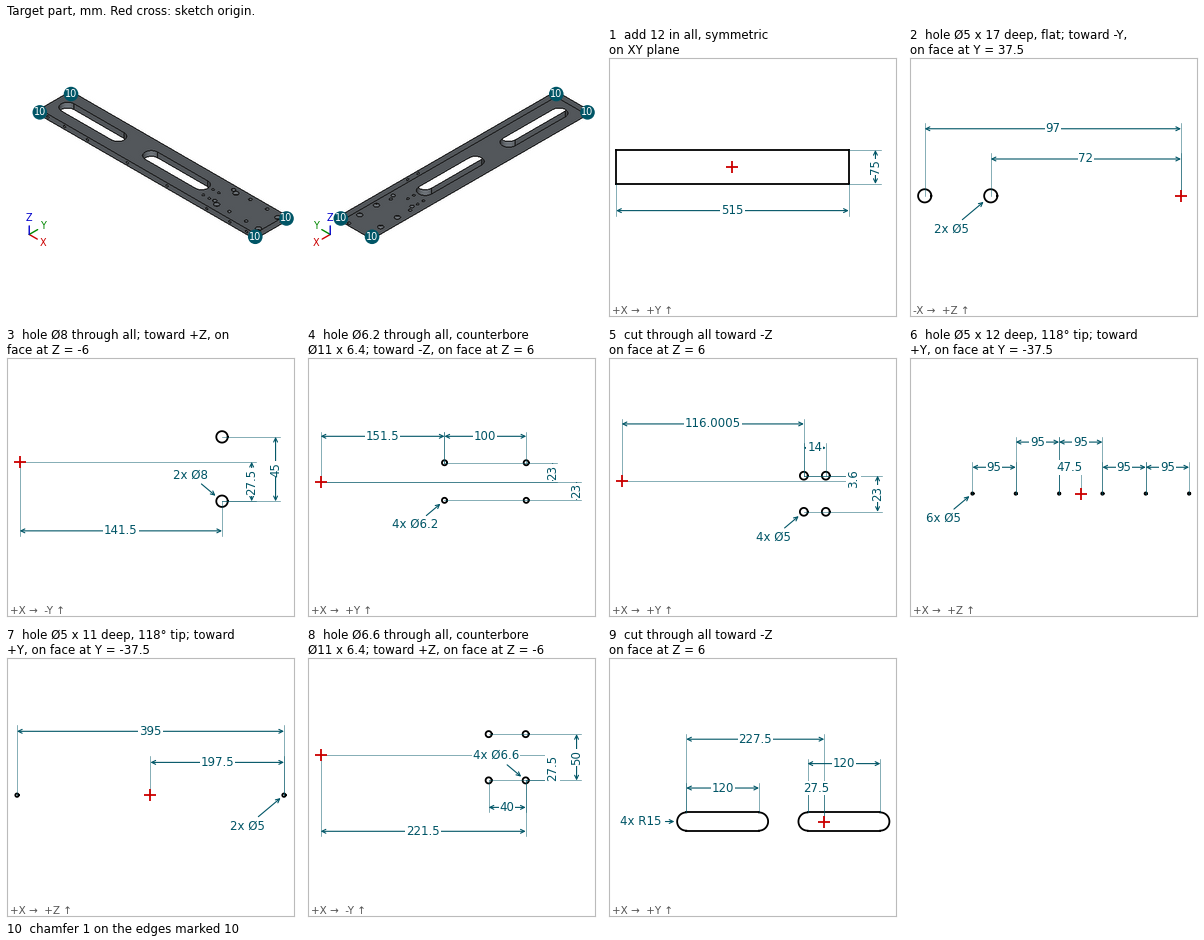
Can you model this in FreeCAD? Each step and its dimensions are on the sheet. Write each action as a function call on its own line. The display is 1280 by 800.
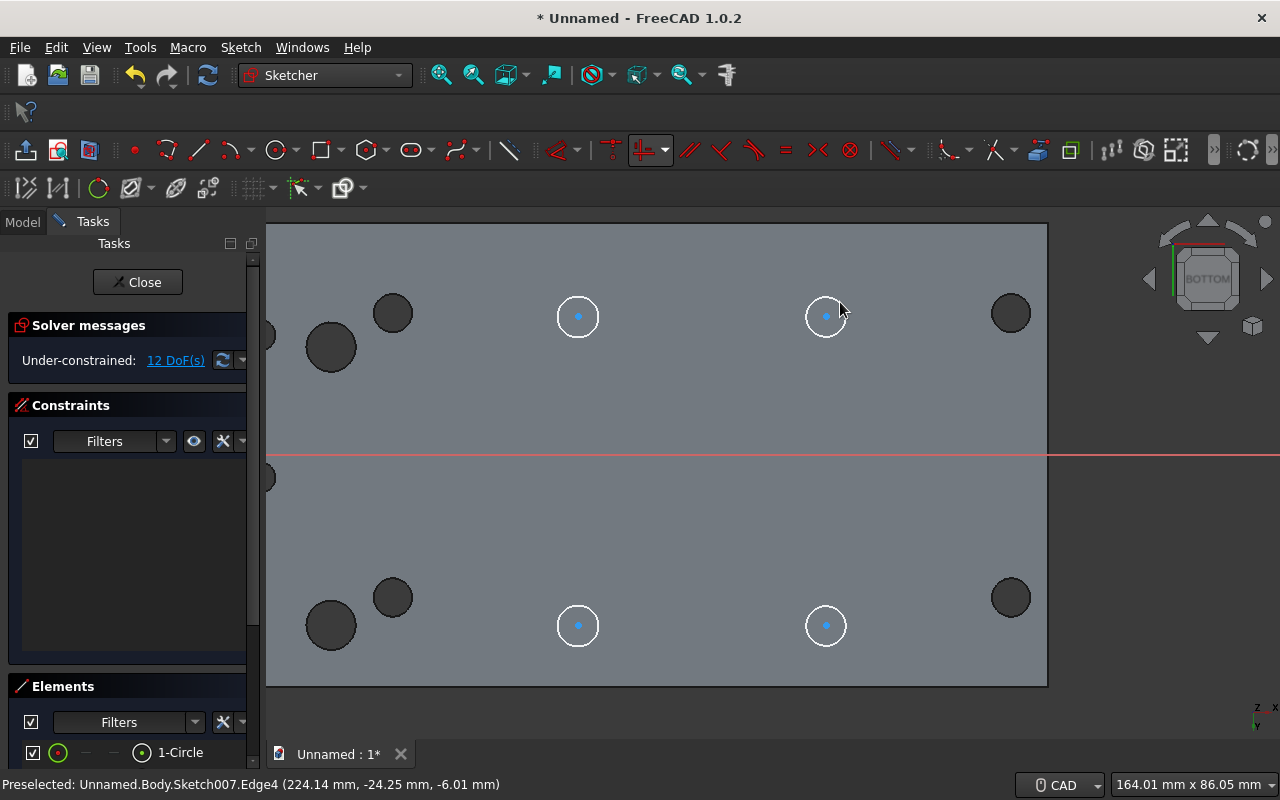
click(840, 612)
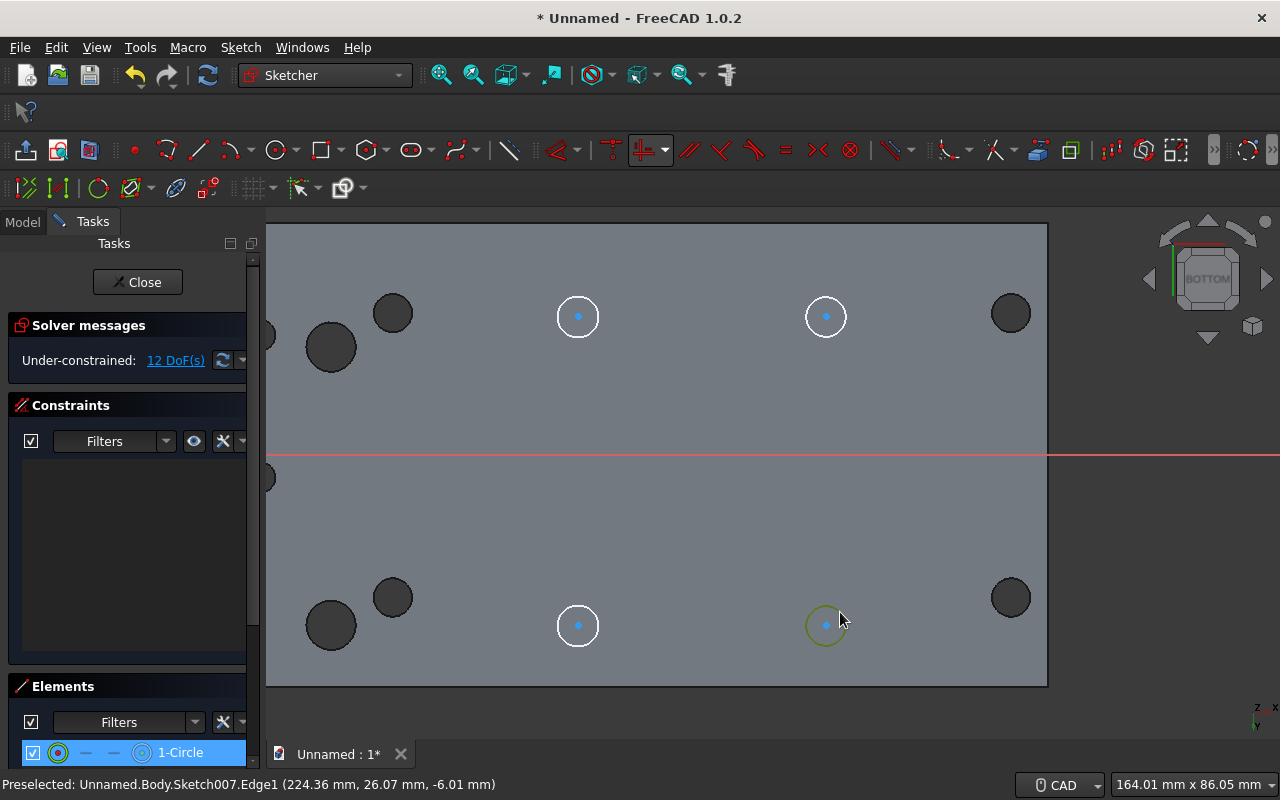
click(592, 611)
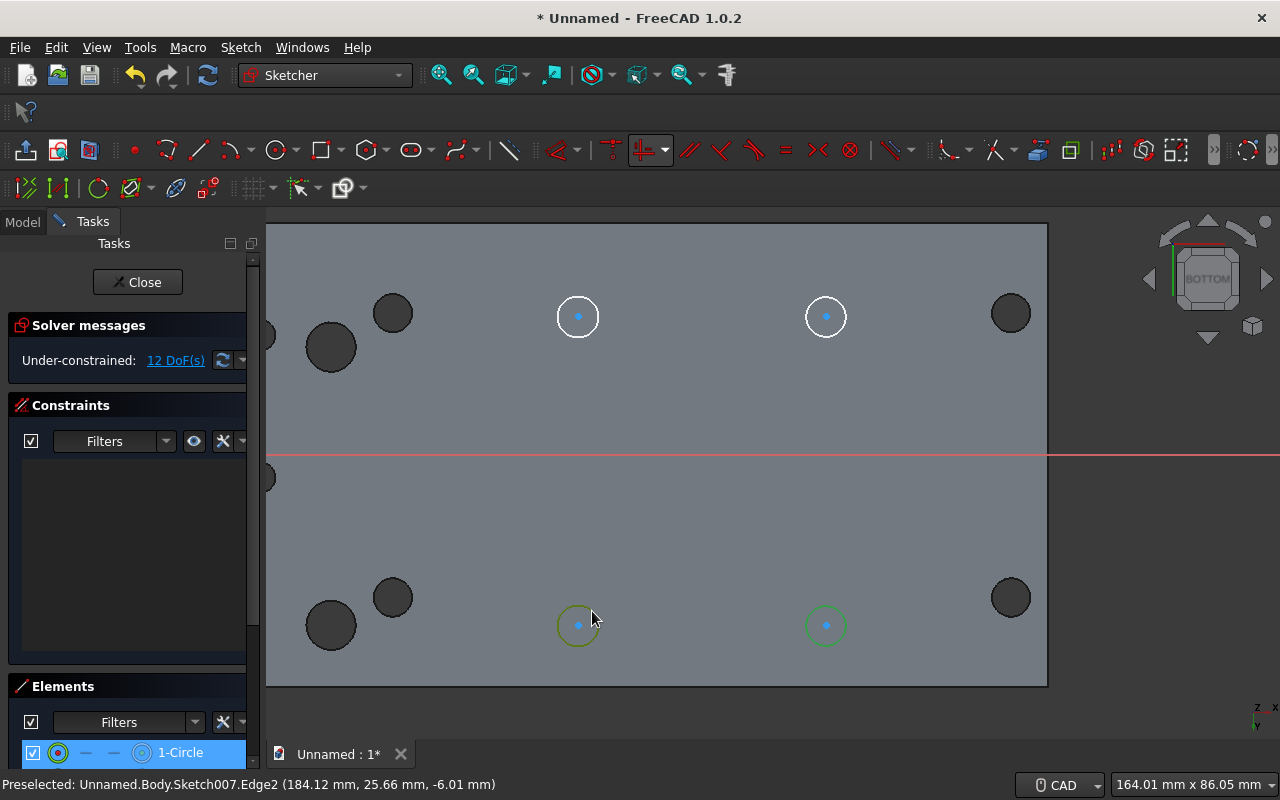
click(592, 302)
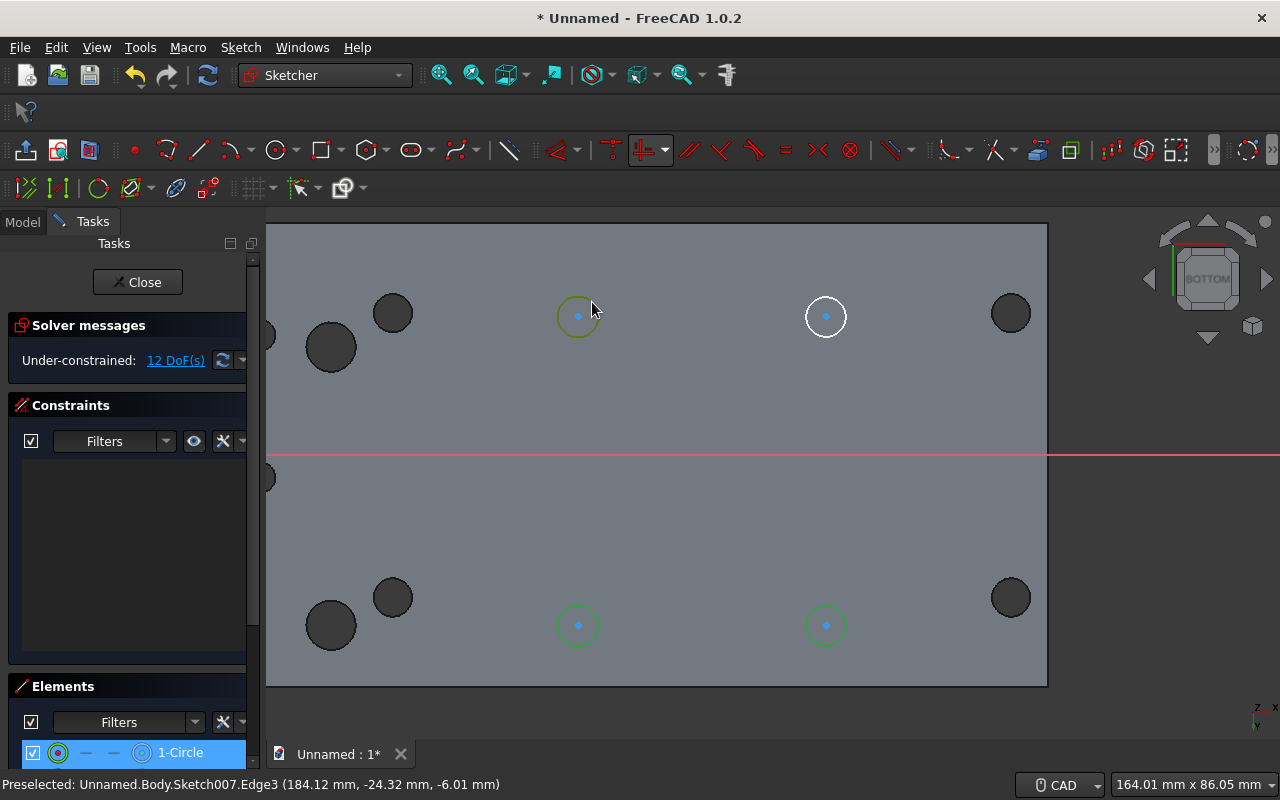
click(840, 303)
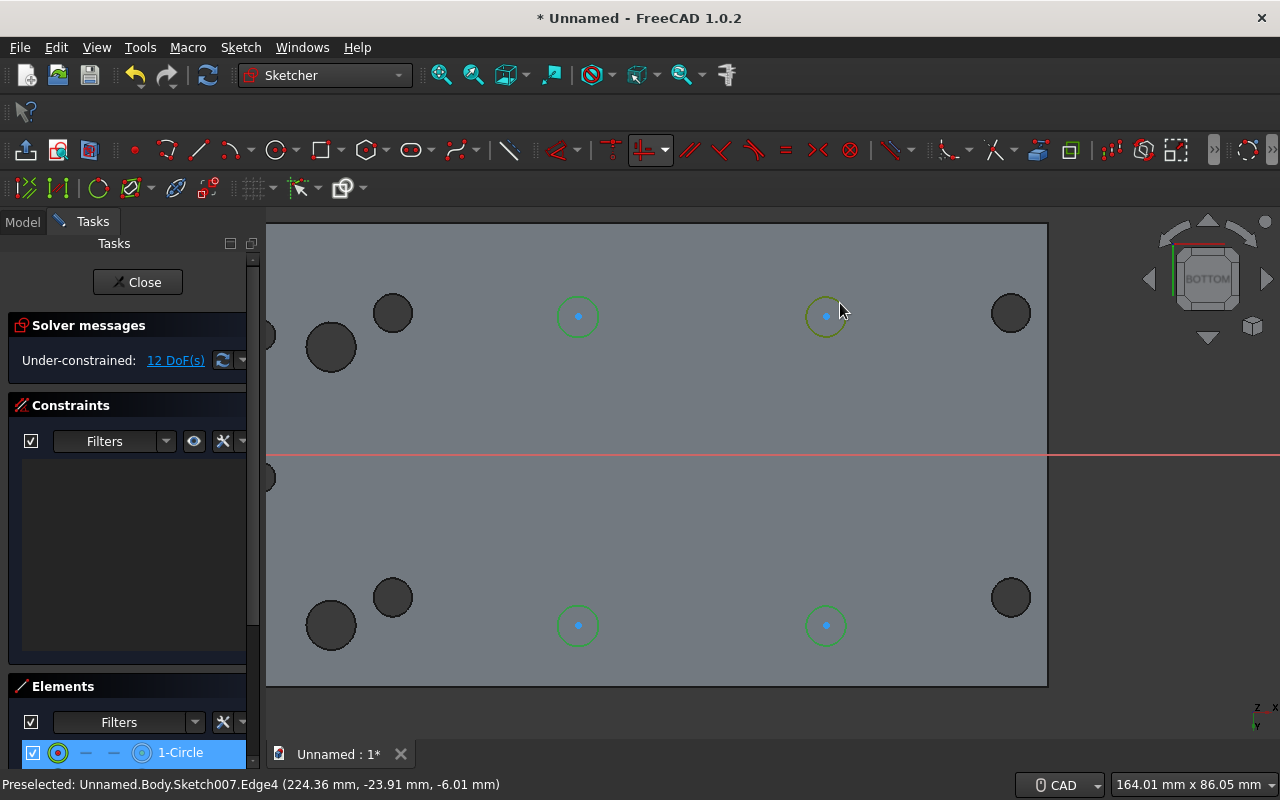
click(786, 150)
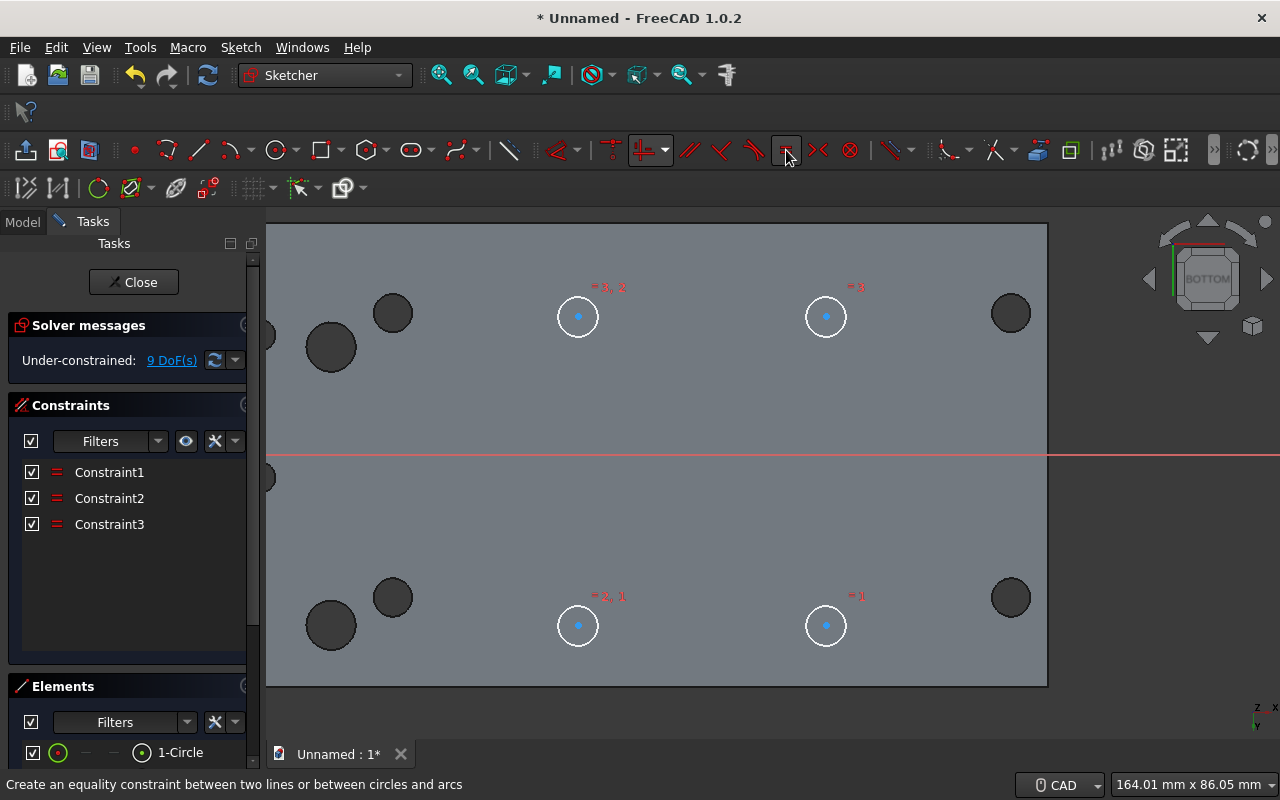
click(826, 626)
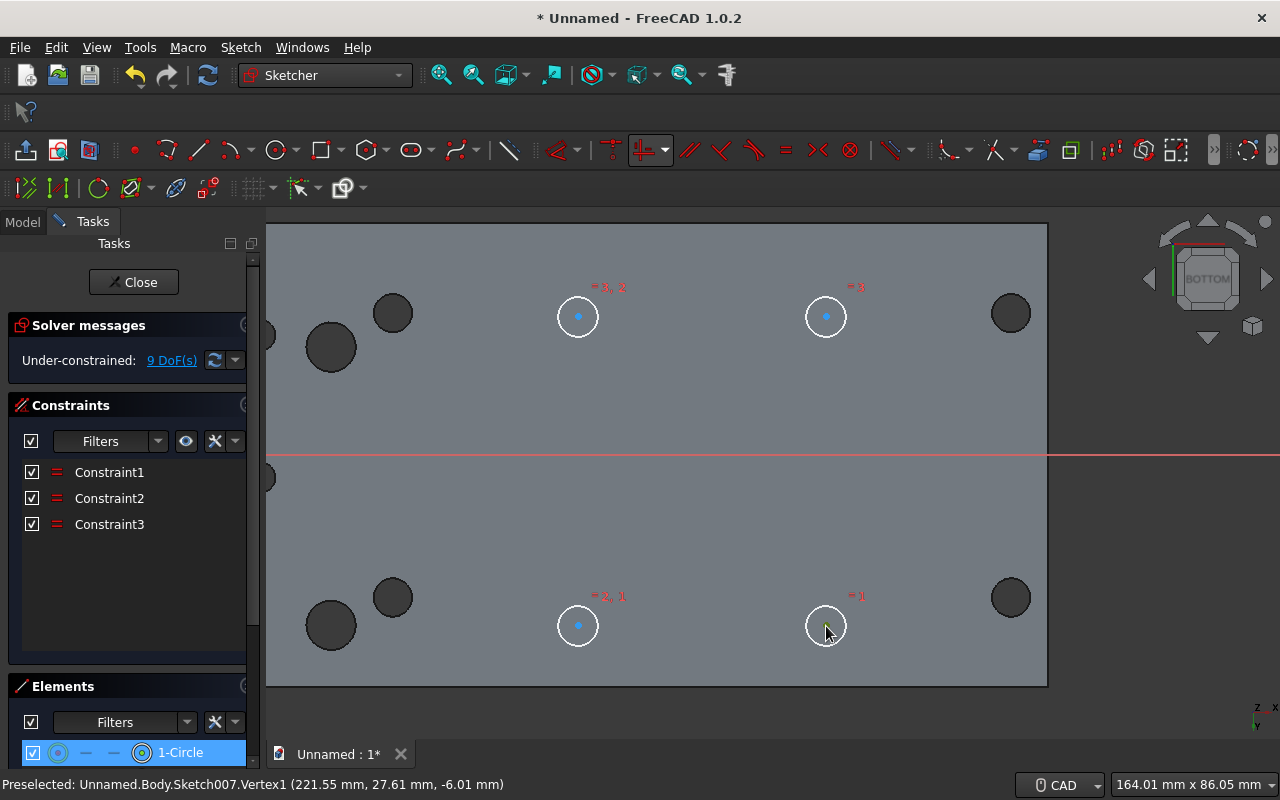
click(578, 626)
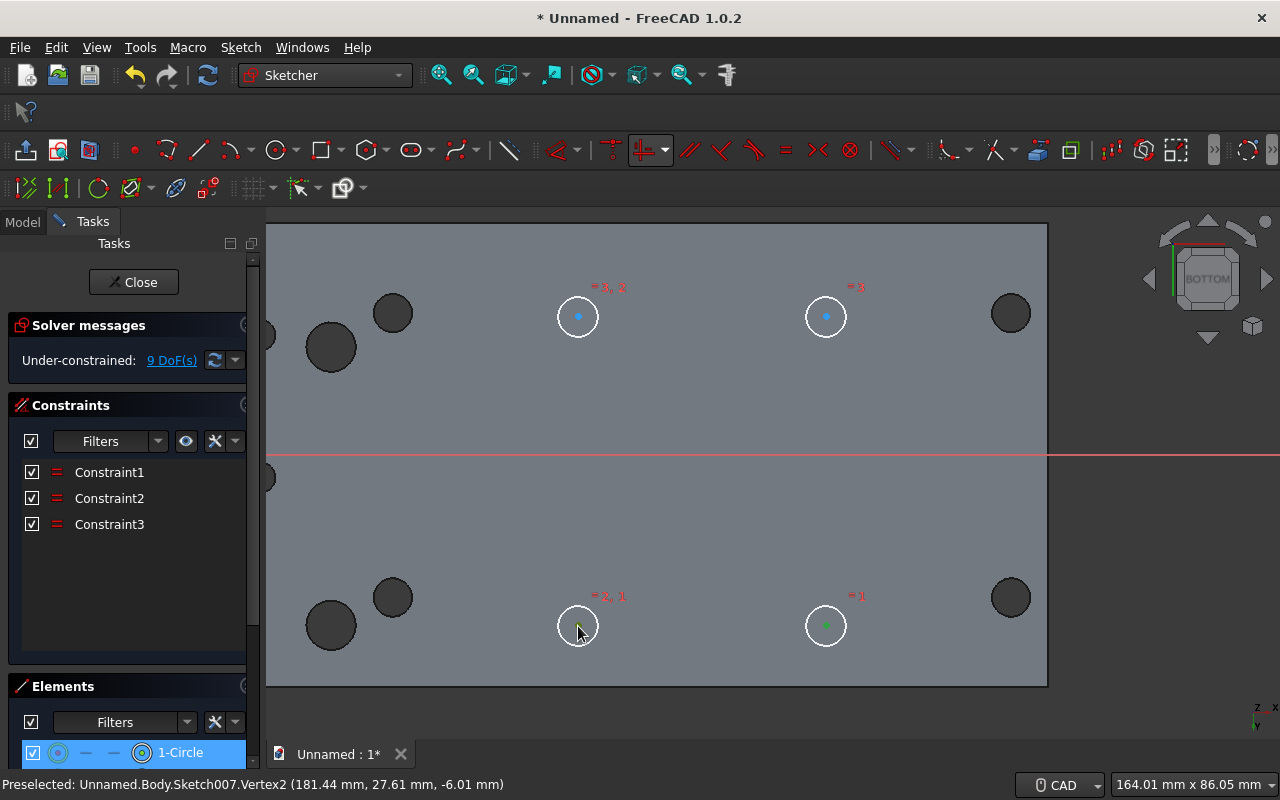
key(h)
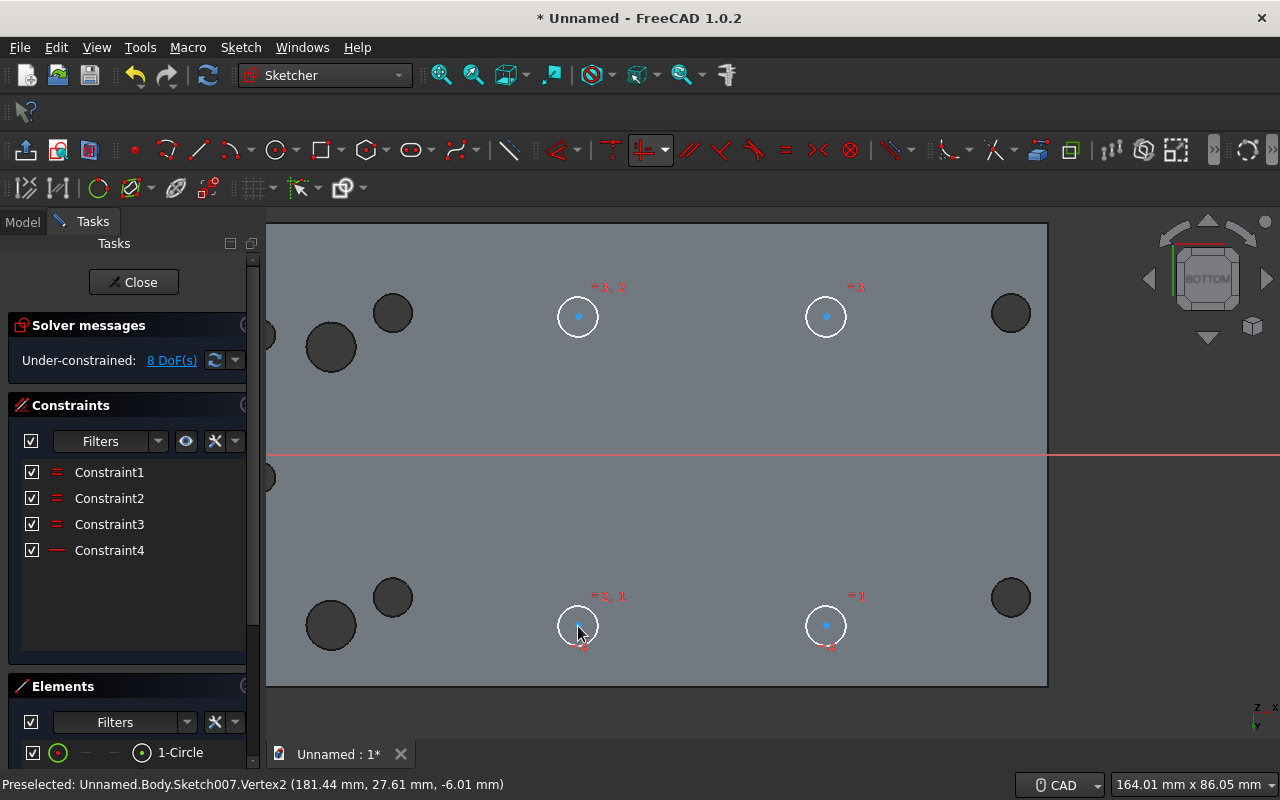
click(578, 626)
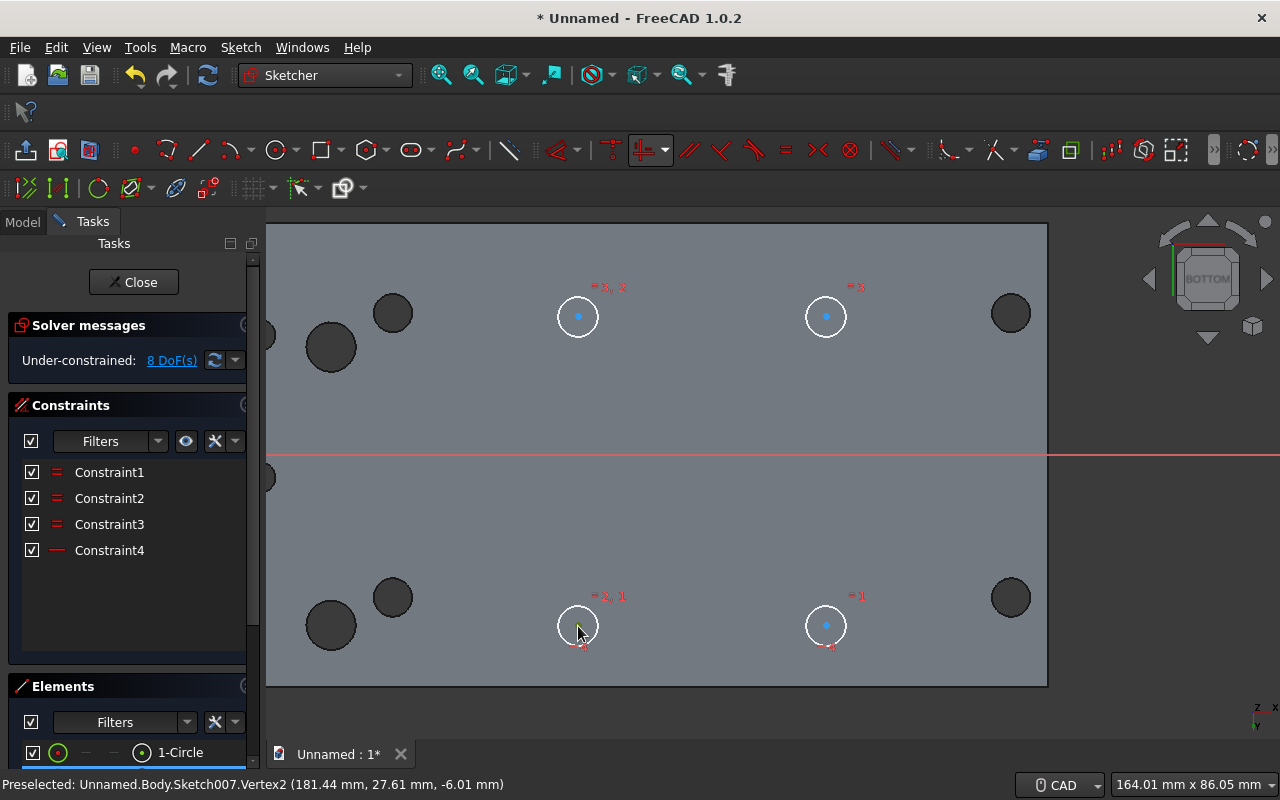
click(578, 317)